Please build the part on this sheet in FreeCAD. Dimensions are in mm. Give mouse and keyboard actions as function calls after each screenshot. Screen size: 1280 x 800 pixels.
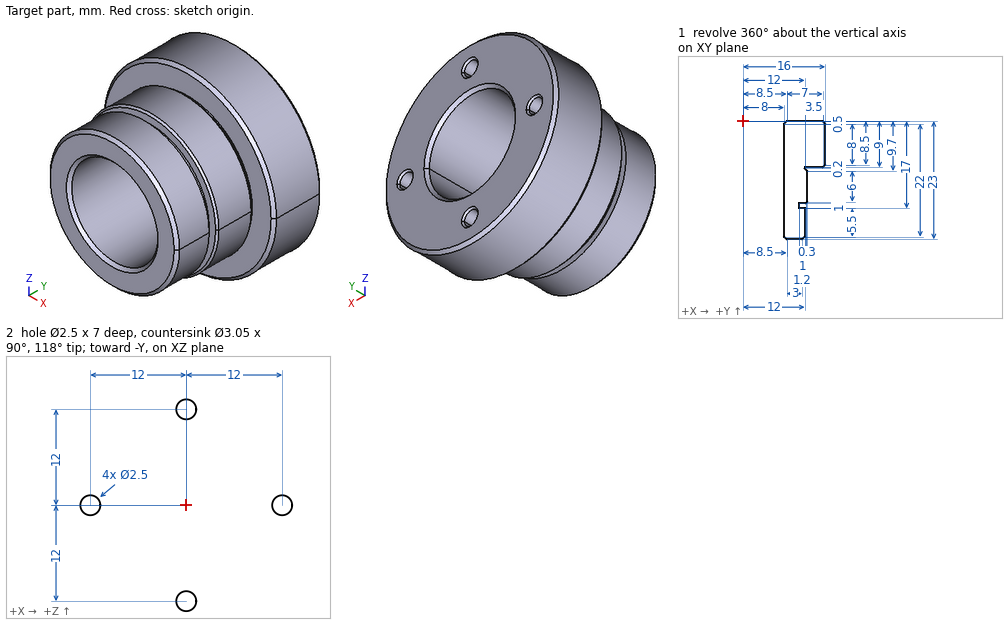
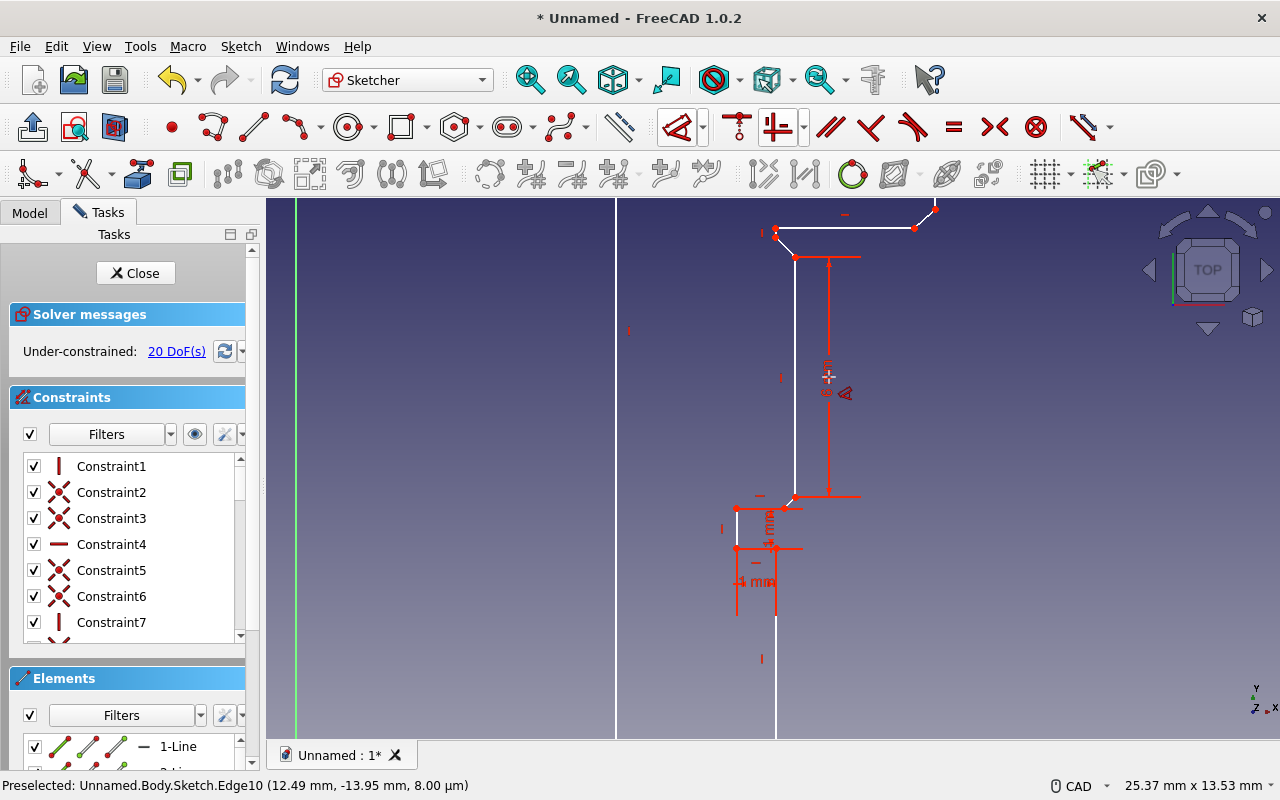
scroll(756, 550, down, 5)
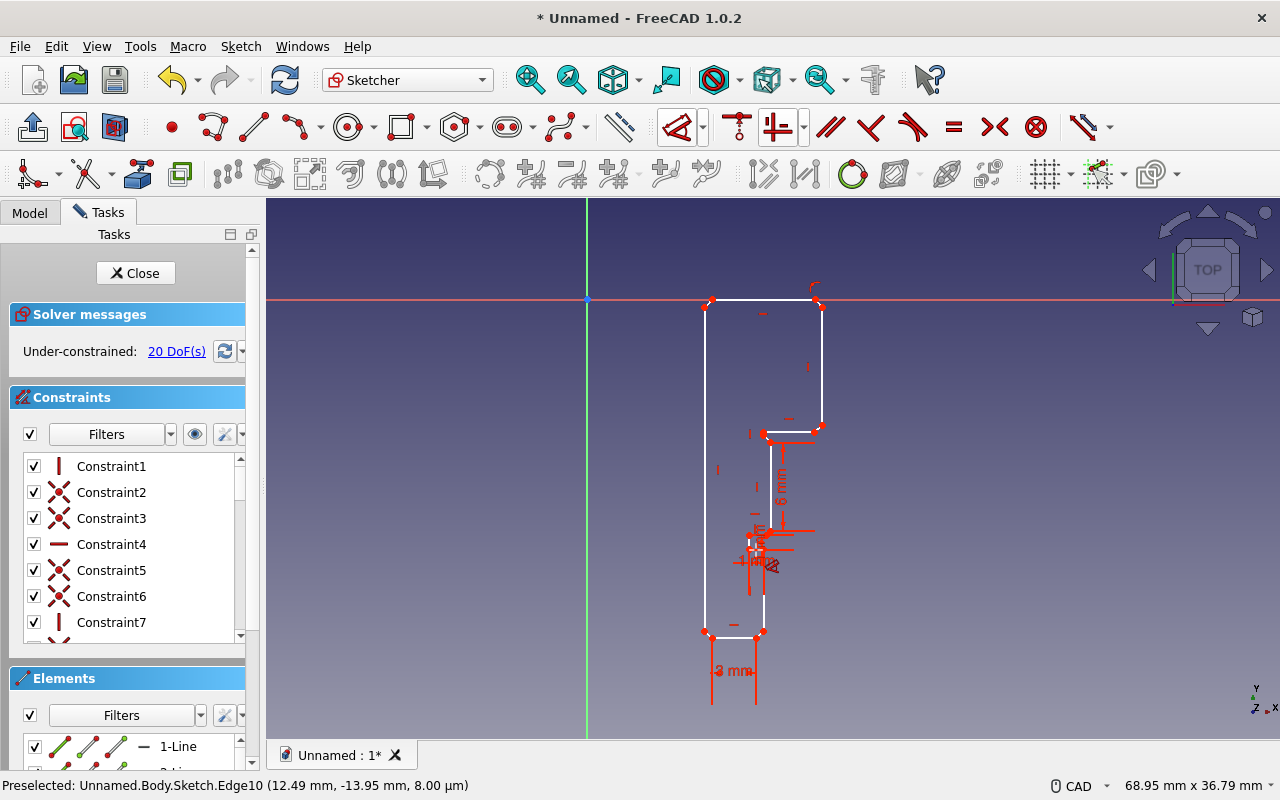
click(822, 390)
click(856, 366)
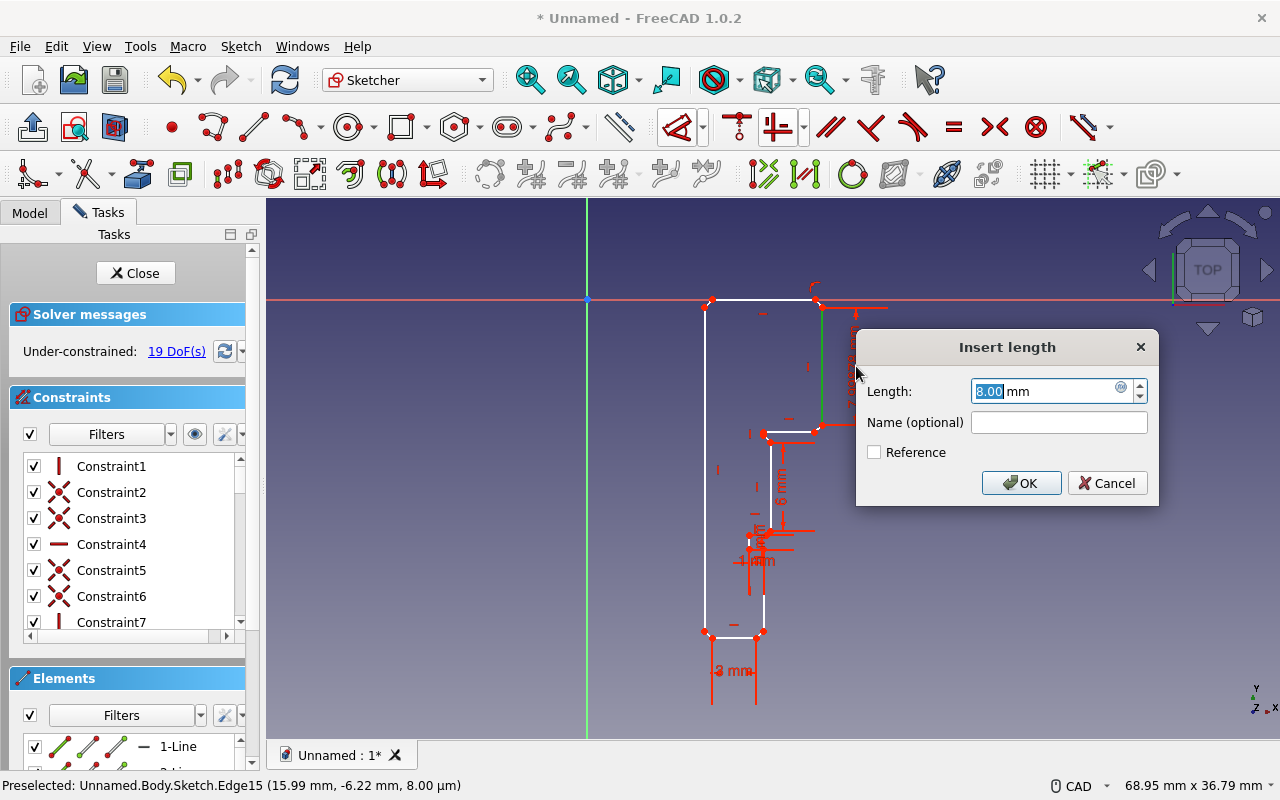
text(8)
key(Return)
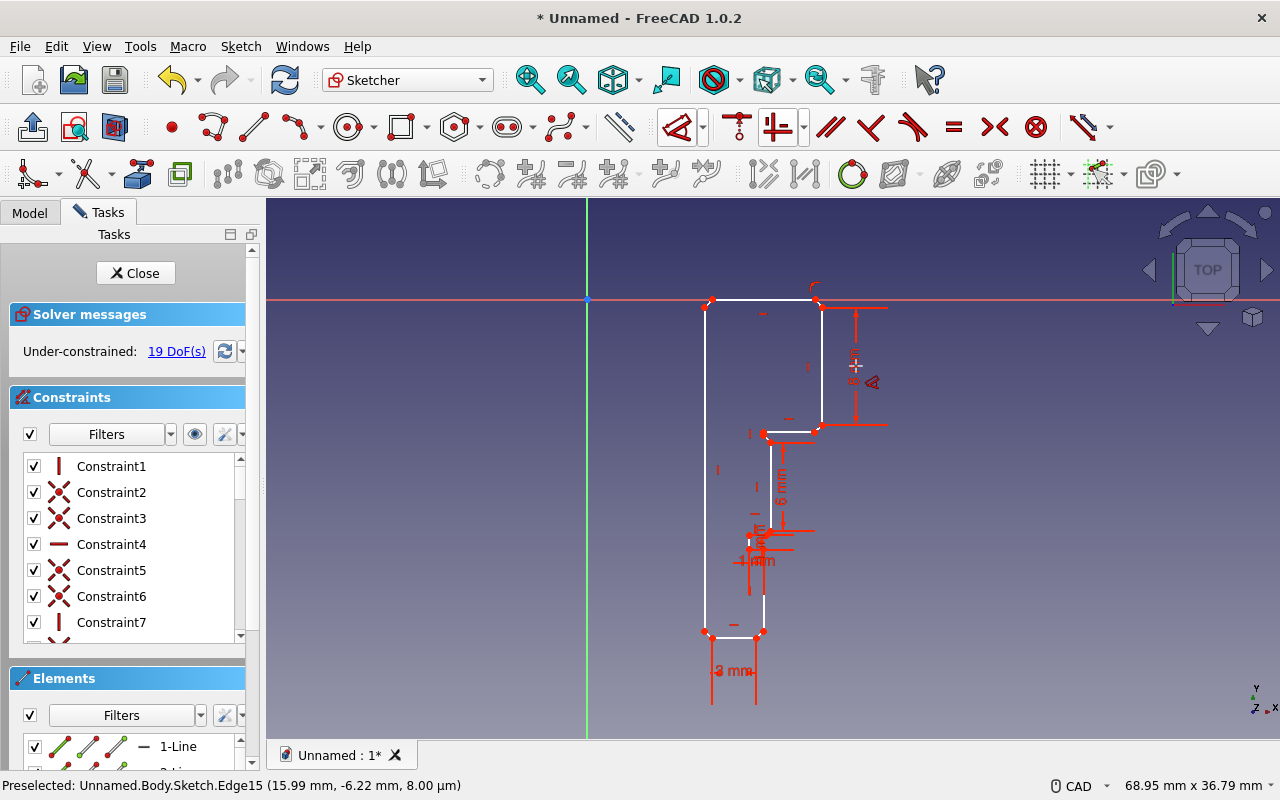
click(784, 300)
click(764, 266)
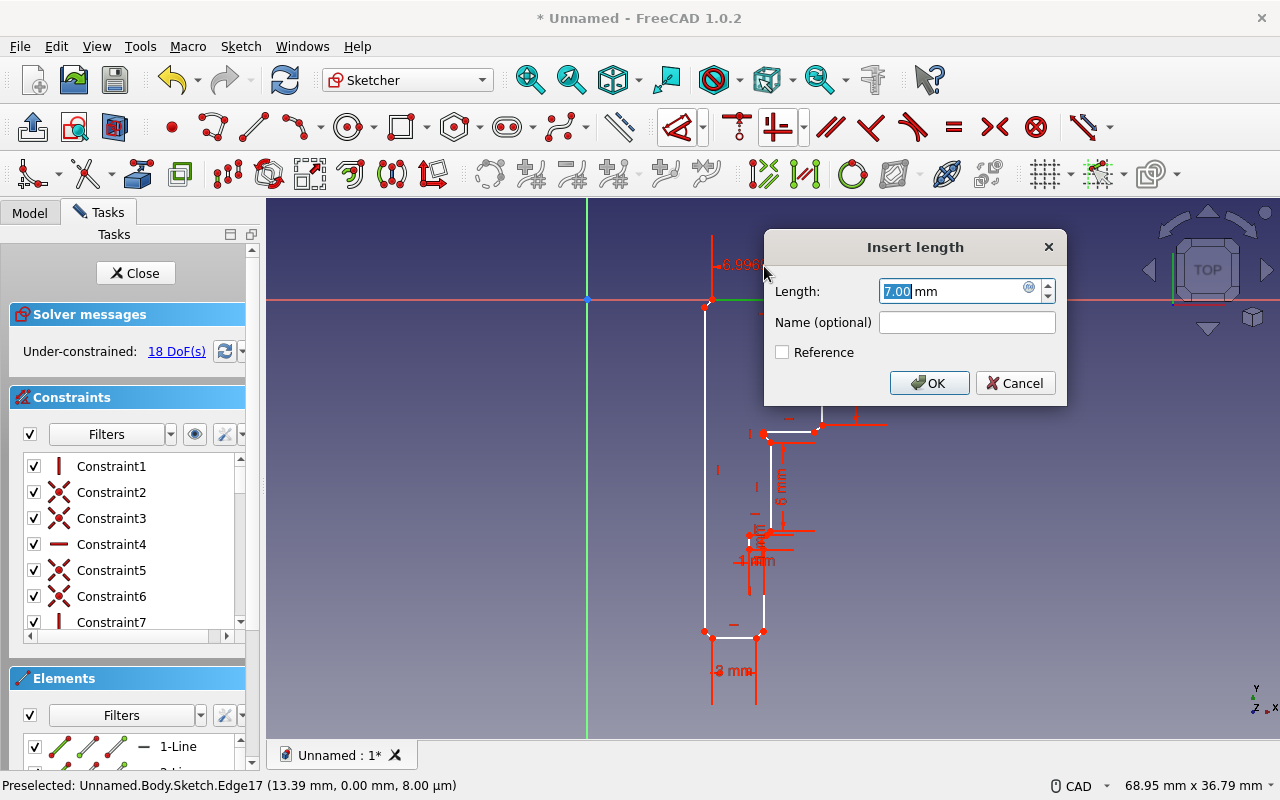
text(7)
key(Return)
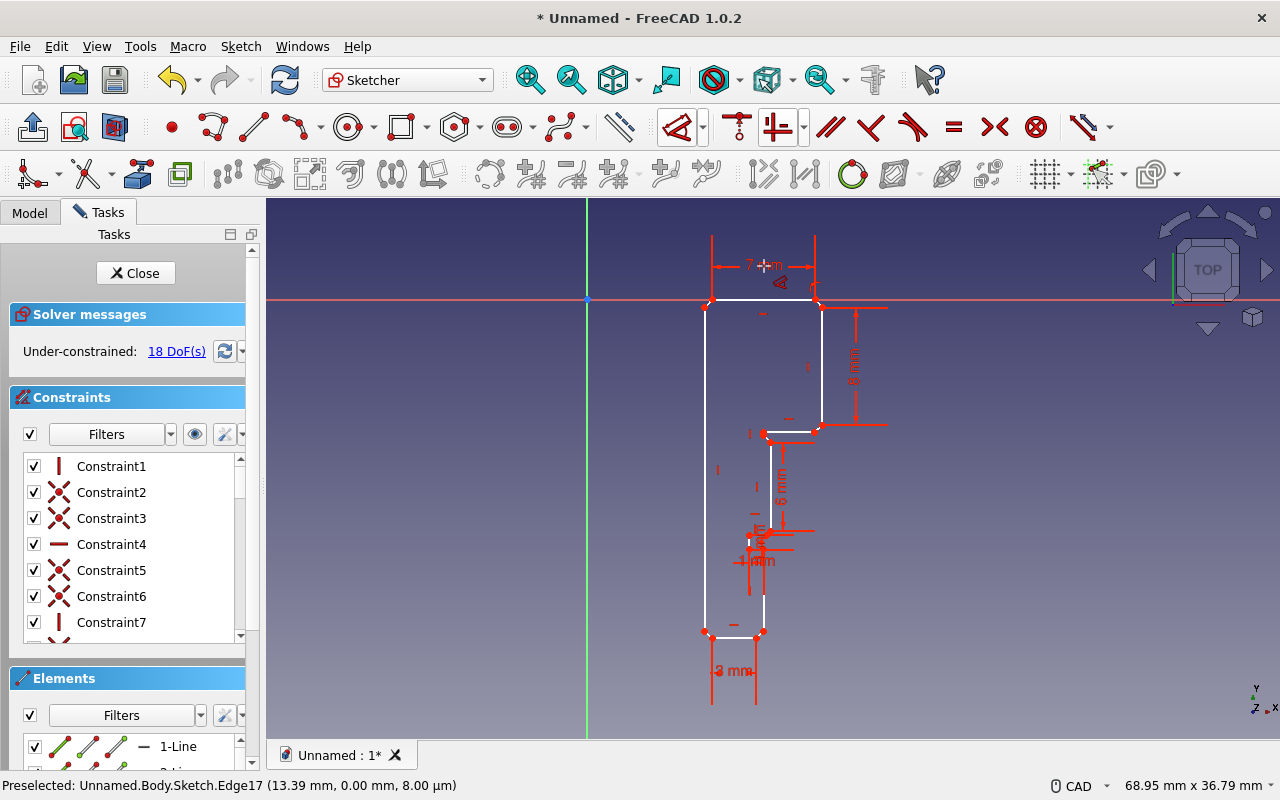
click(705, 405)
click(739, 395)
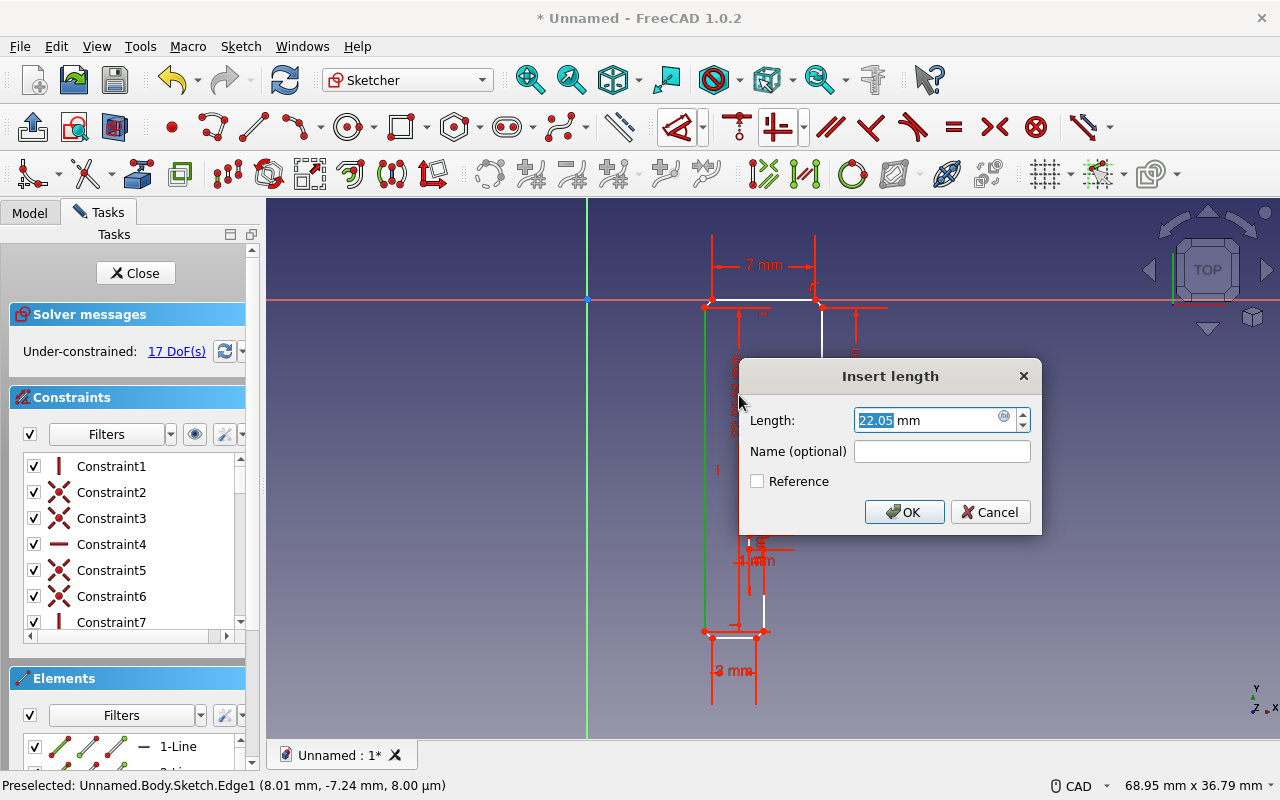
text(22)
key(Return)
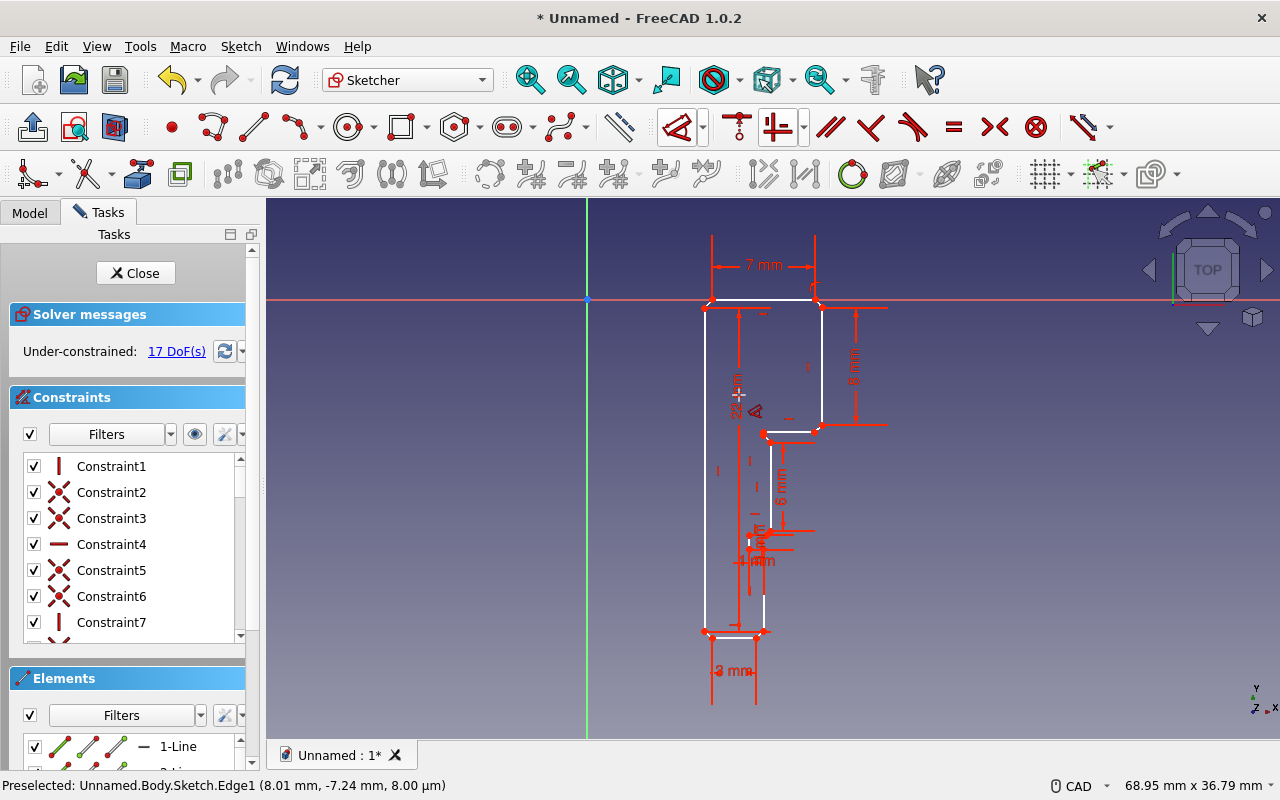
click(705, 308)
click(646, 266)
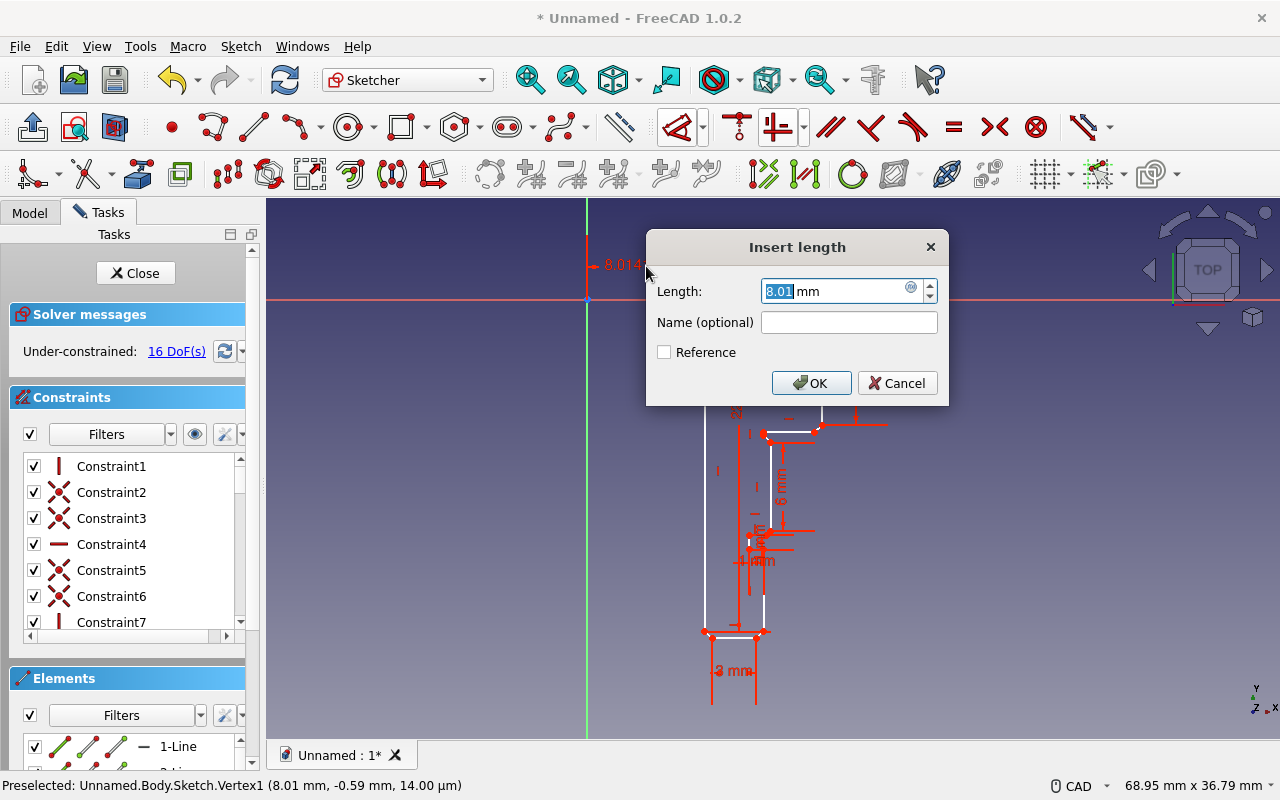
text(8)
key(Return)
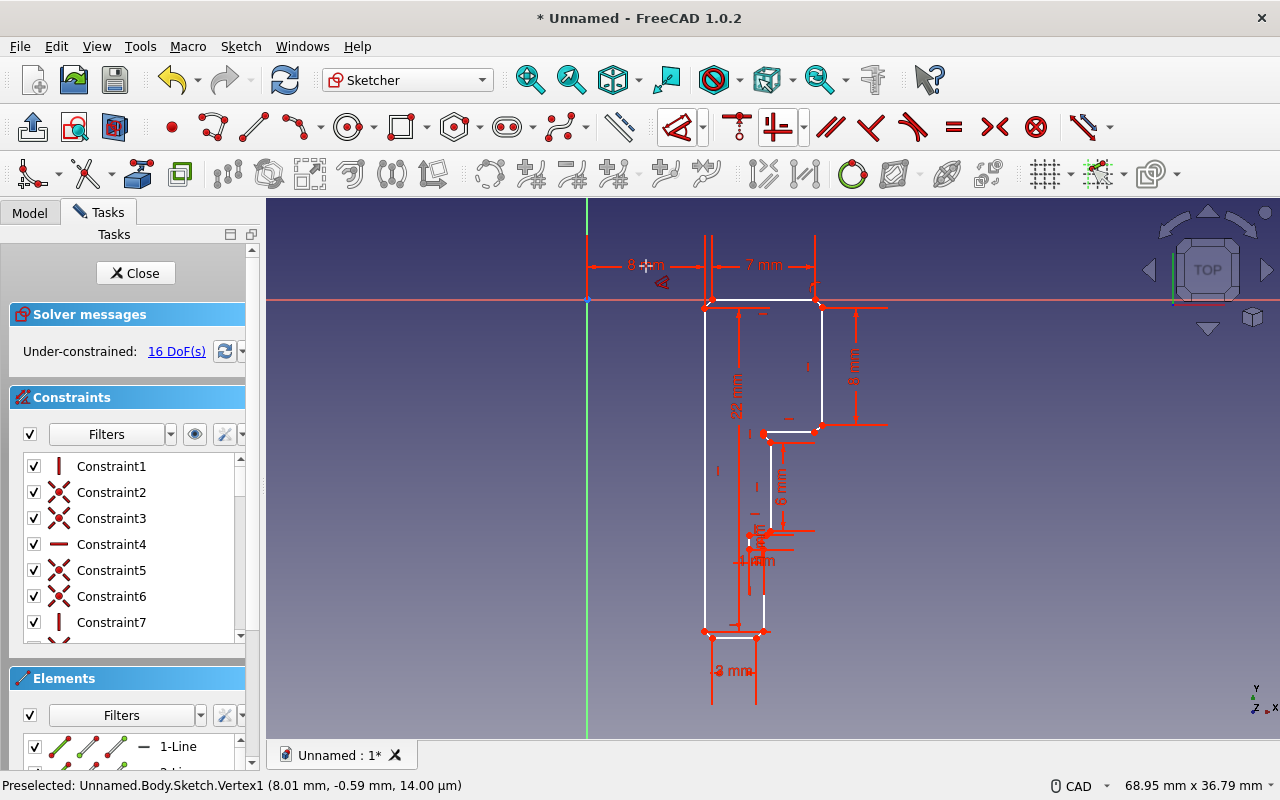
scroll(764, 432, up, 7)